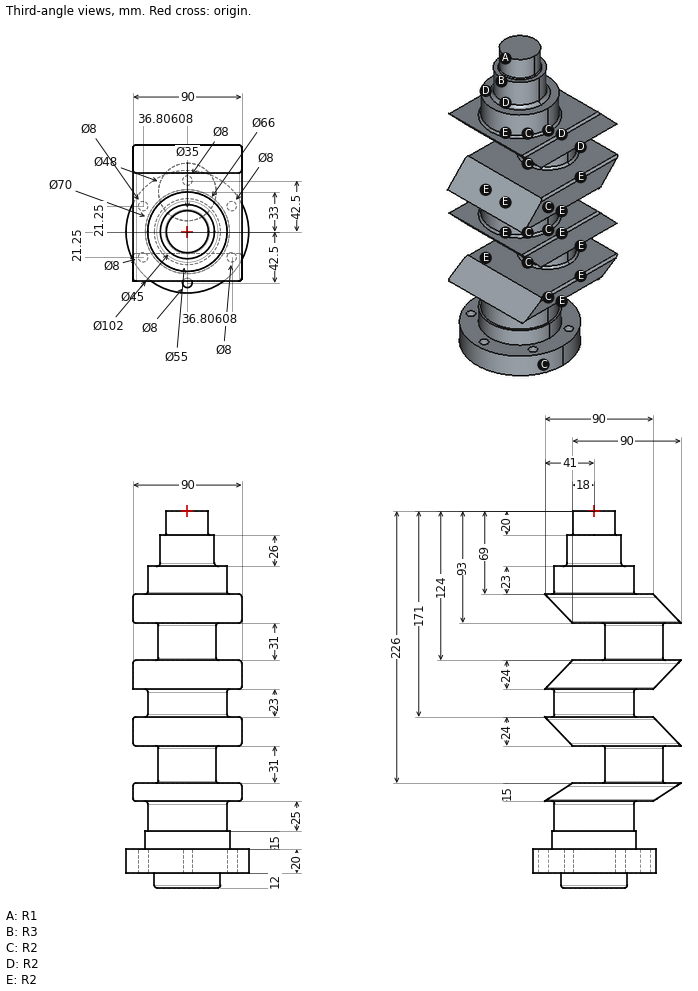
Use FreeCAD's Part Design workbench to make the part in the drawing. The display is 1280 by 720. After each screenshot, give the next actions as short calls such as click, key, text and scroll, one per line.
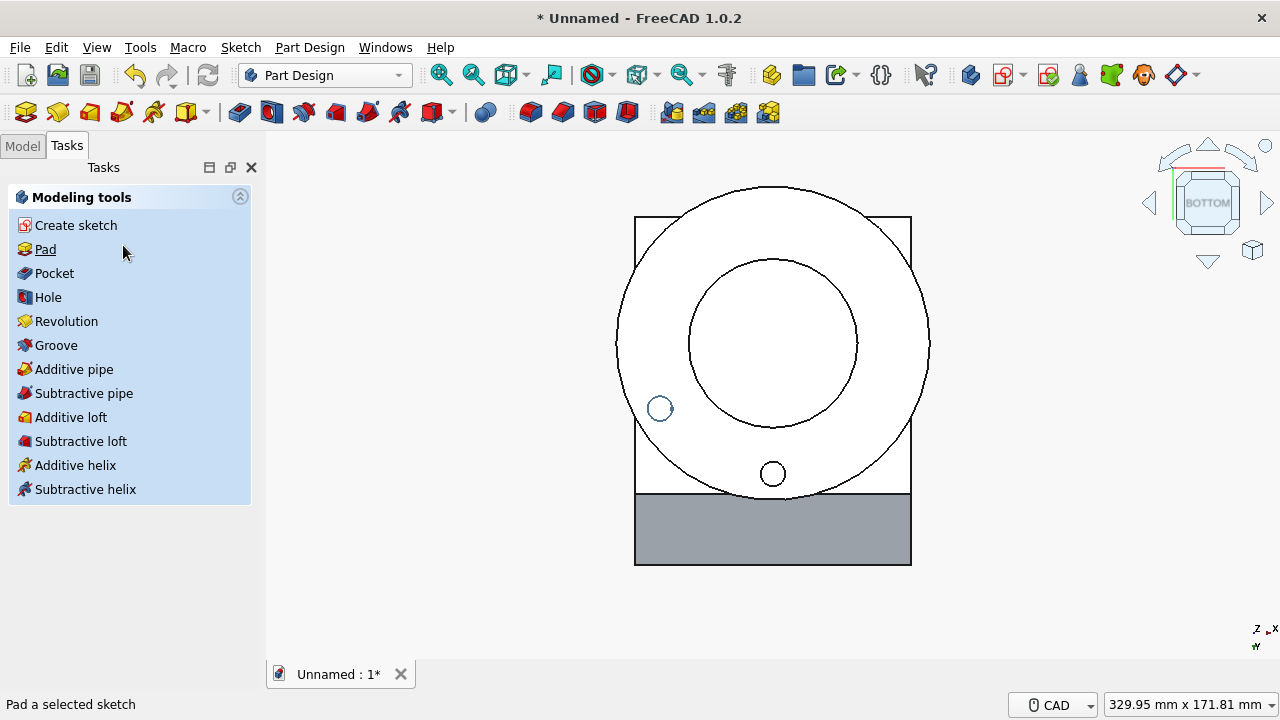
click(240, 112)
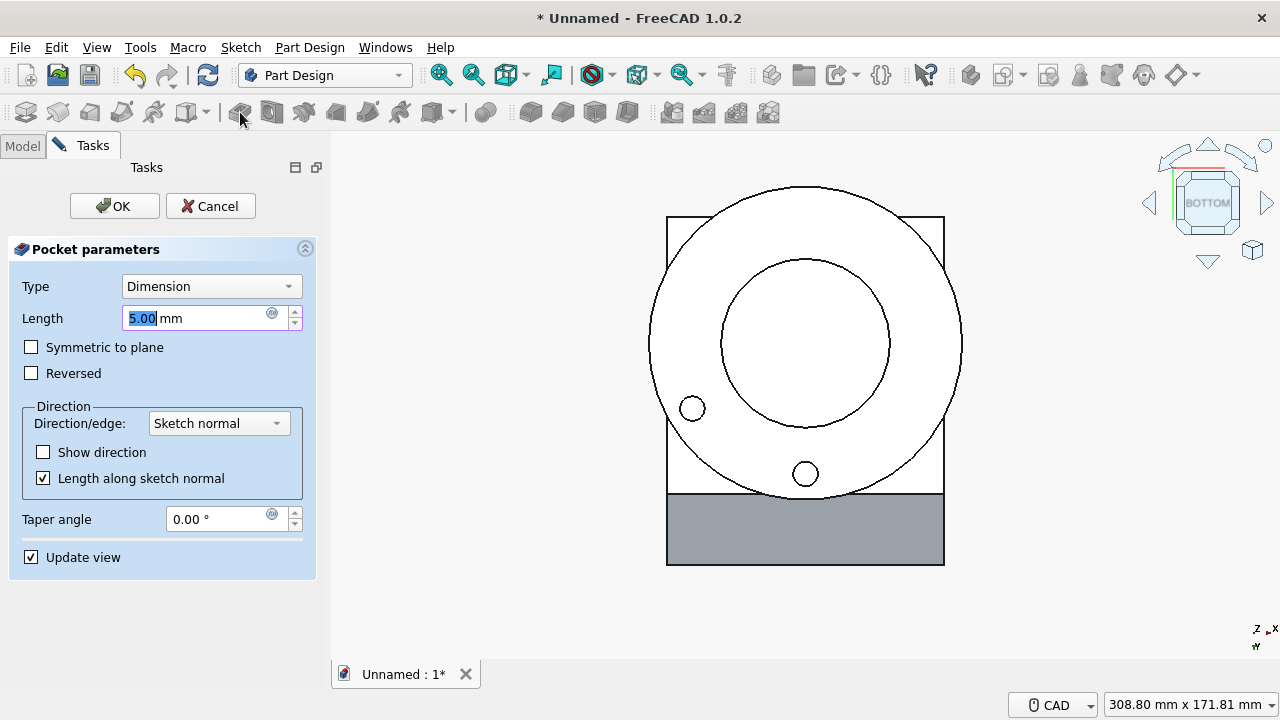
click(212, 286)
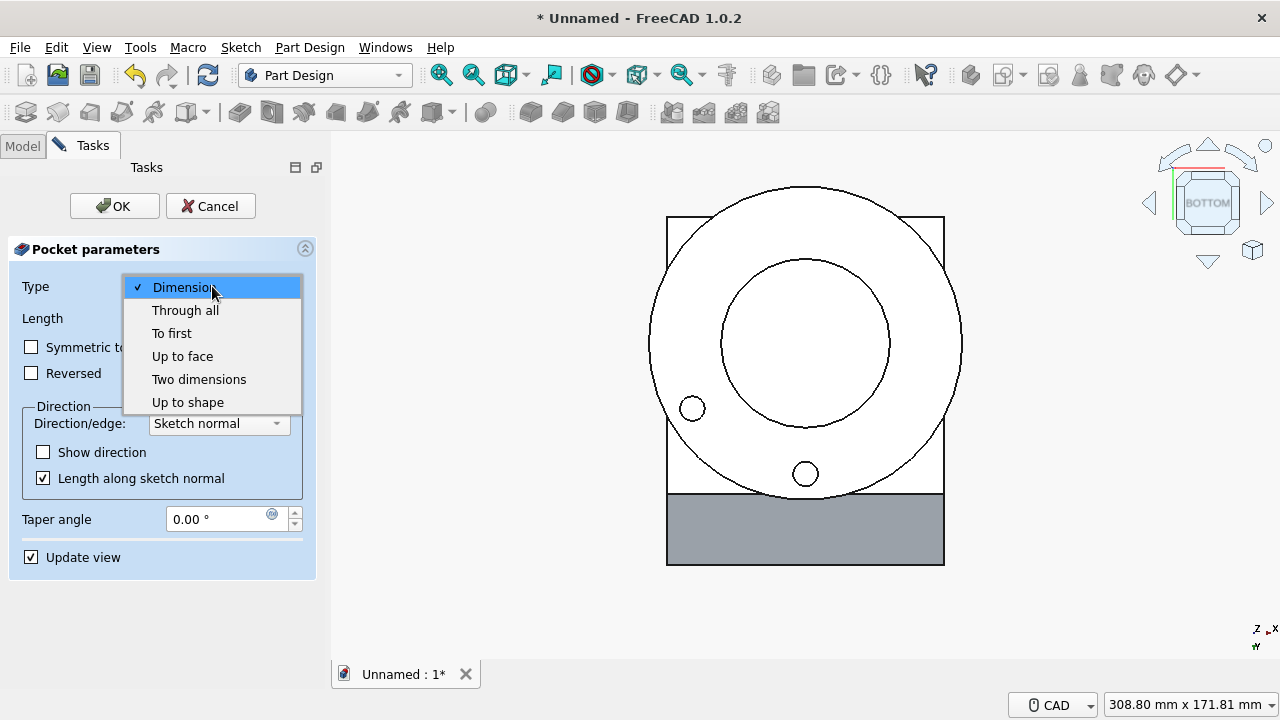
click(212, 334)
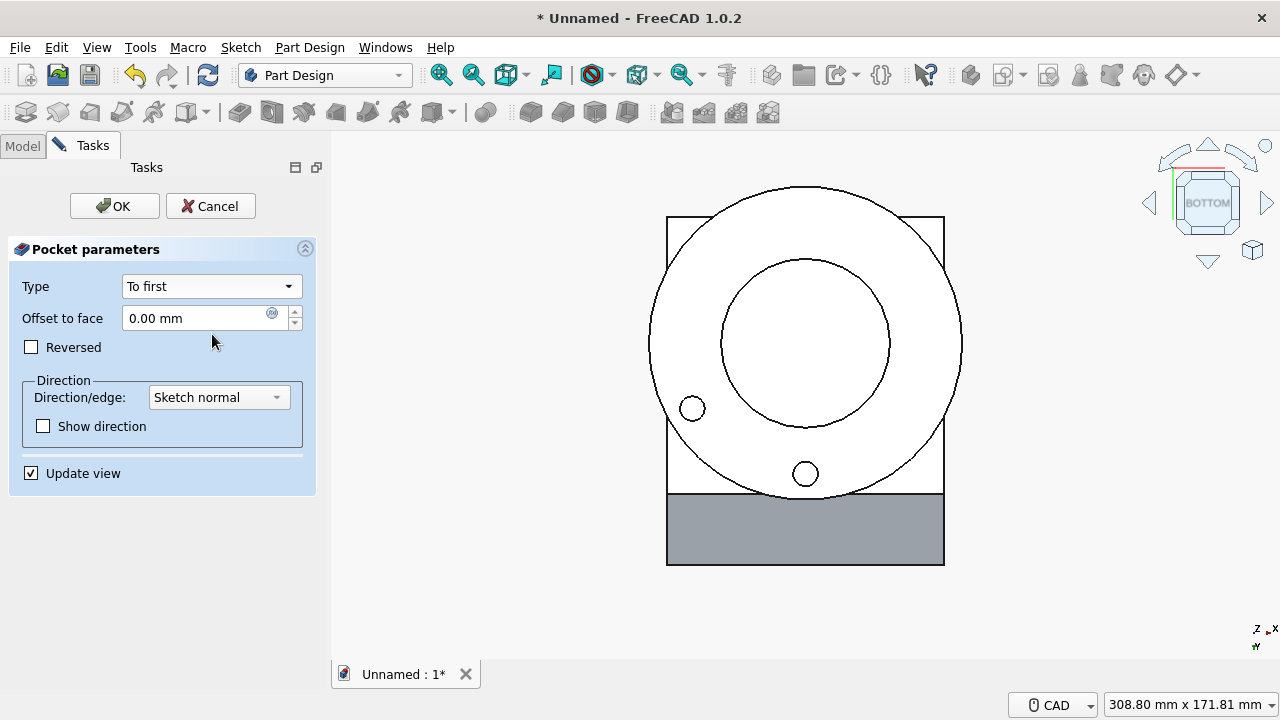
click(115, 206)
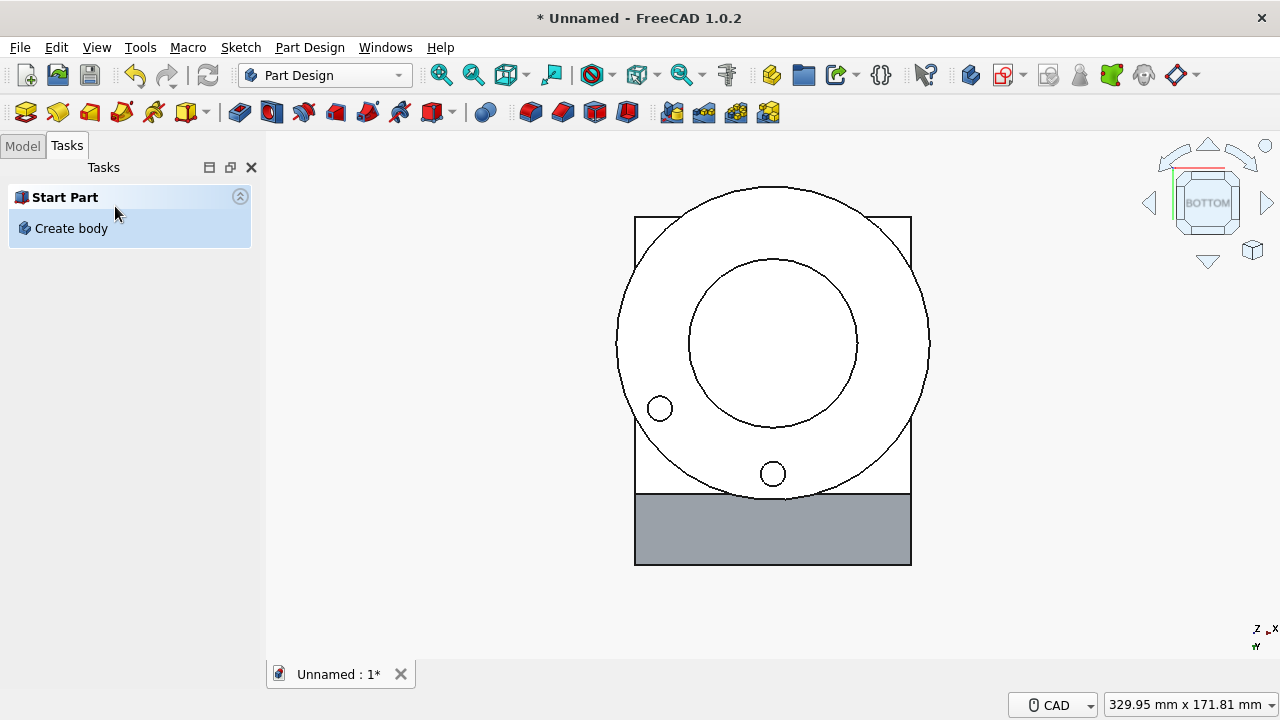
click(863, 432)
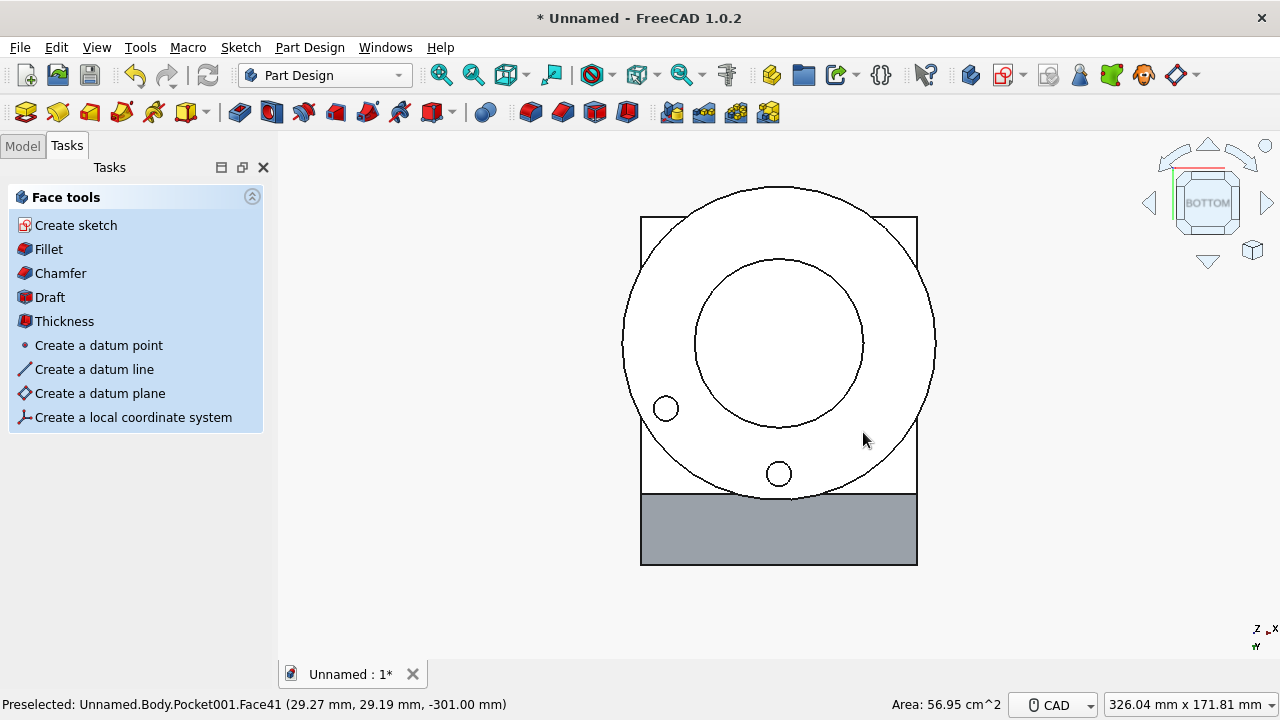
click(1004, 76)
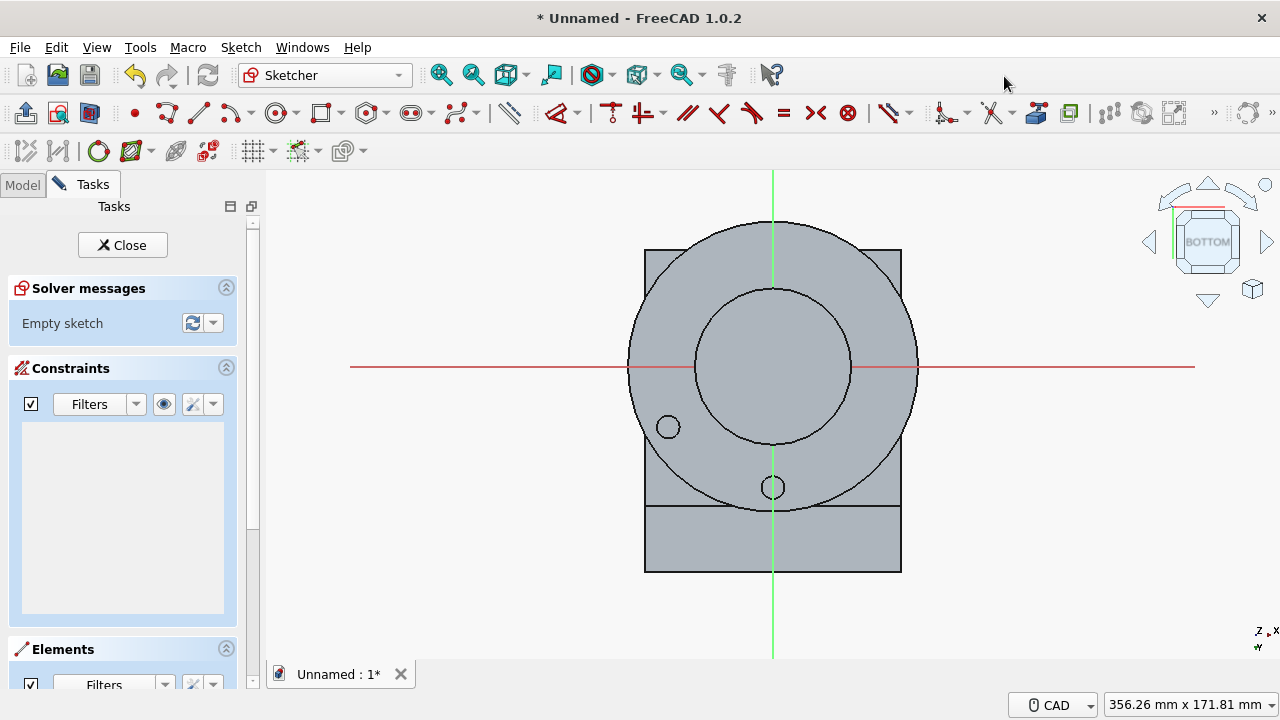
click(90, 114)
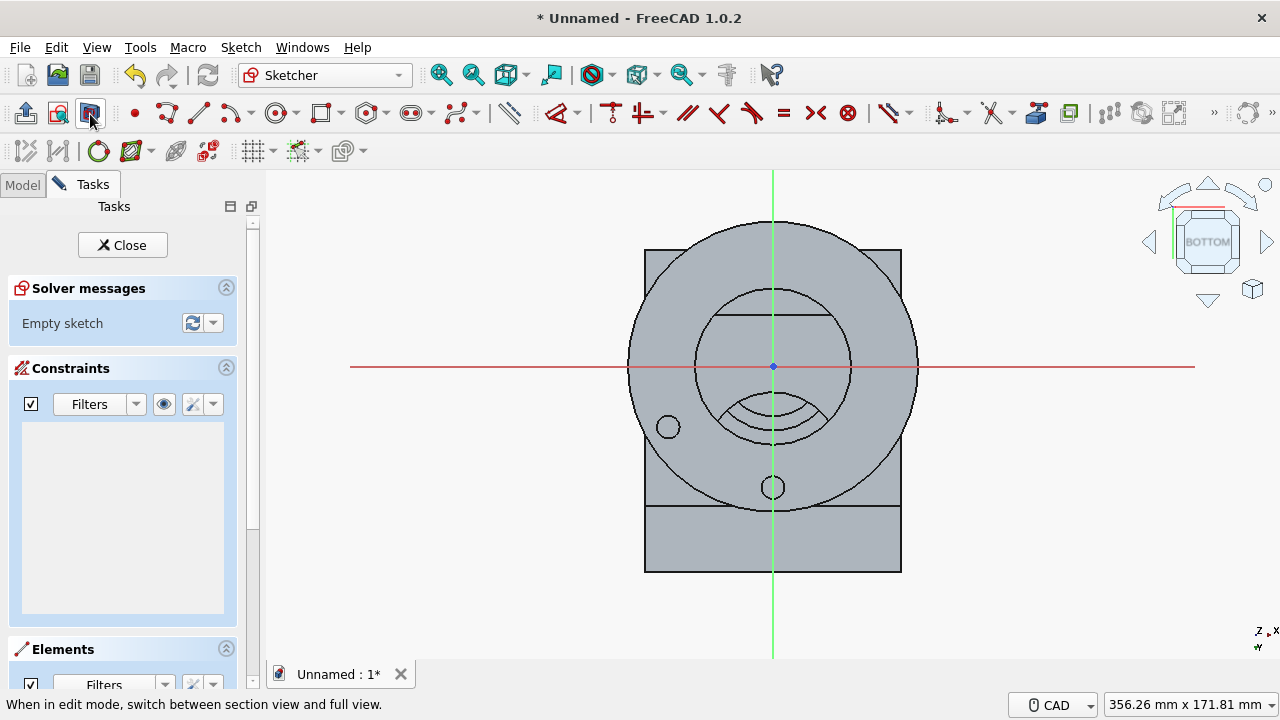
scroll(665, 297, up, 13)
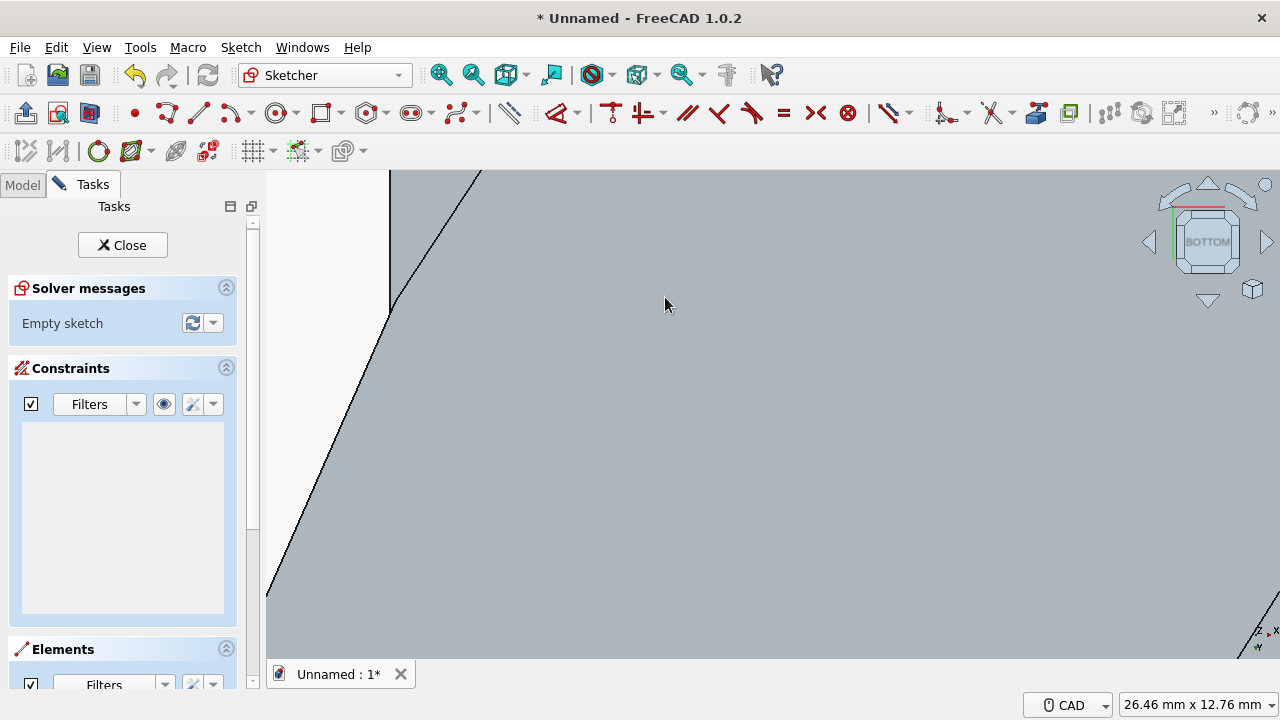
click(276, 114)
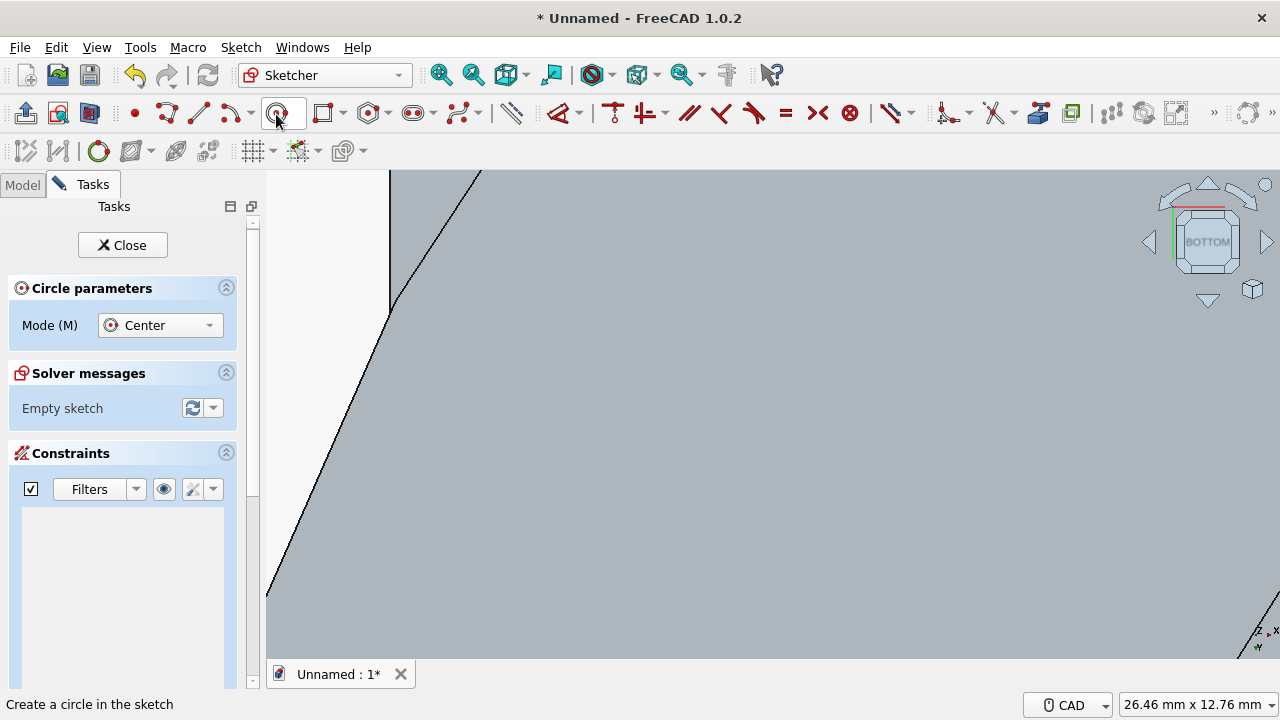
click(704, 417)
move(813, 308)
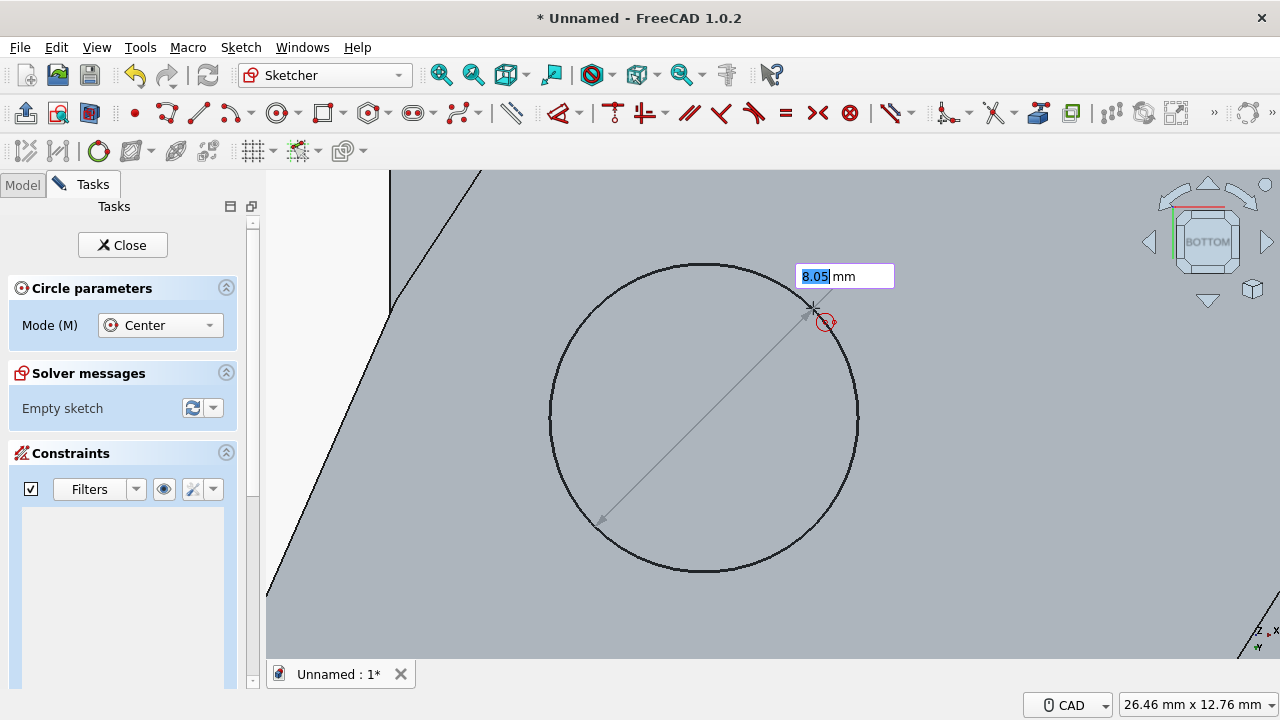
text(8)
key(Return)
key(Escape)